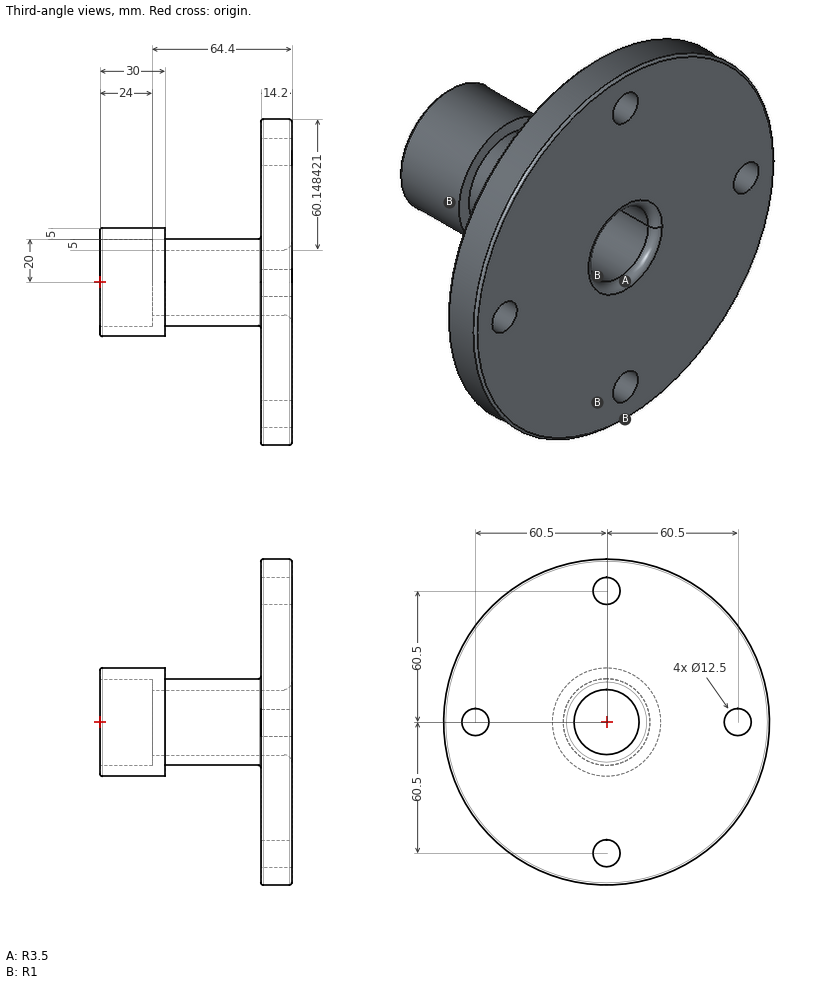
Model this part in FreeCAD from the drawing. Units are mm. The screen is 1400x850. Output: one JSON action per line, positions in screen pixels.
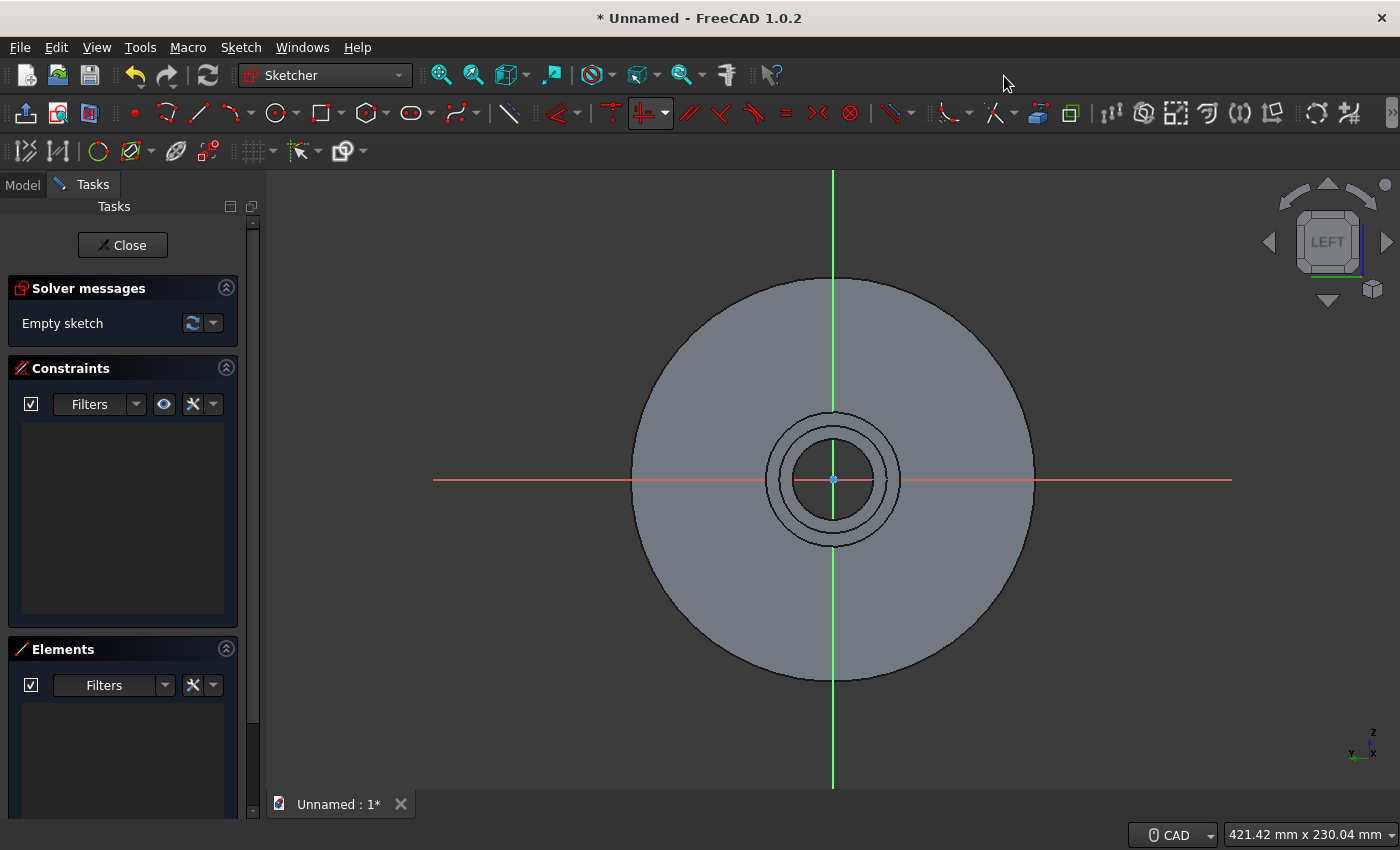
{"action": "key", "text": "q s"}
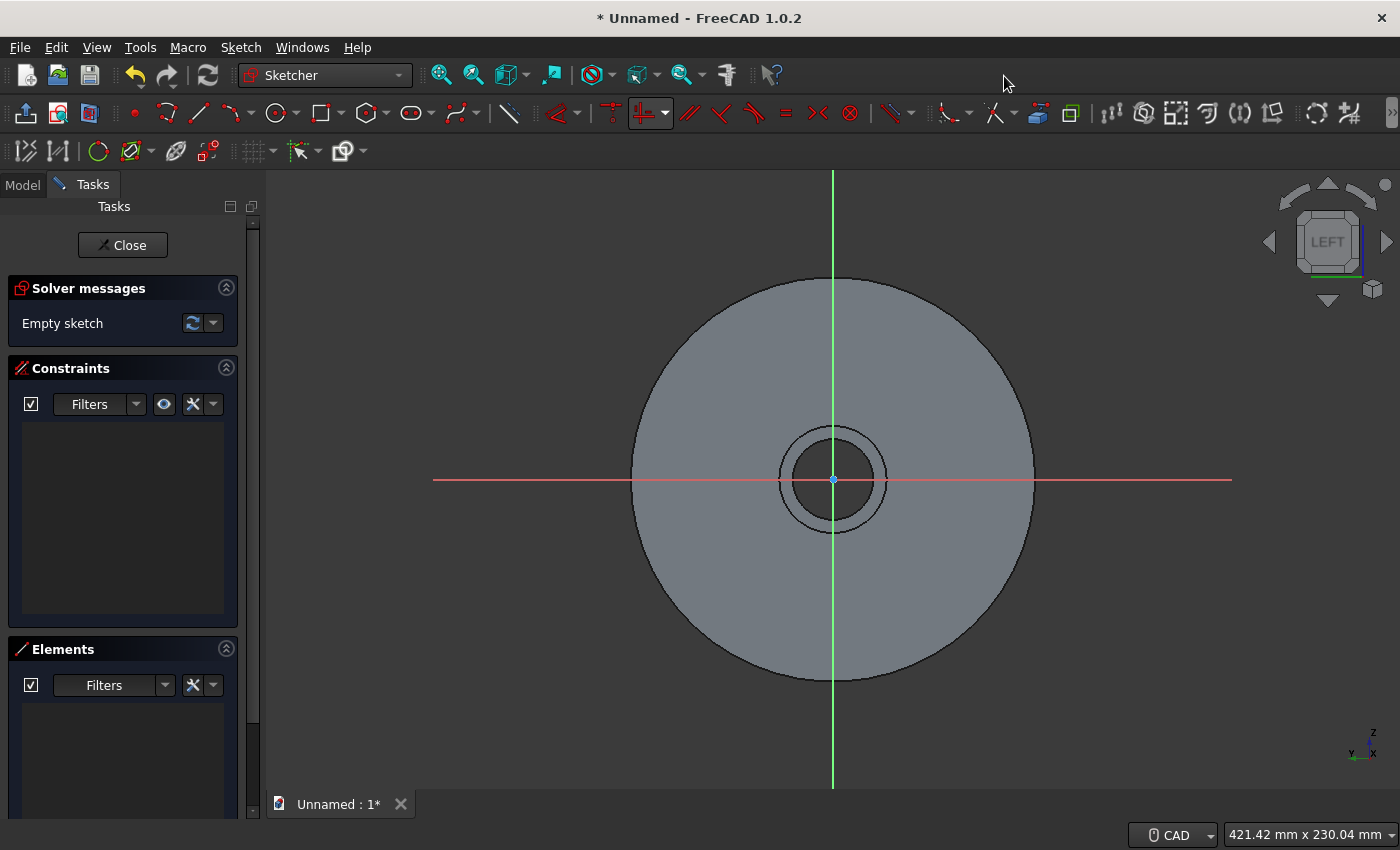
{"action": "key", "text": "g c"}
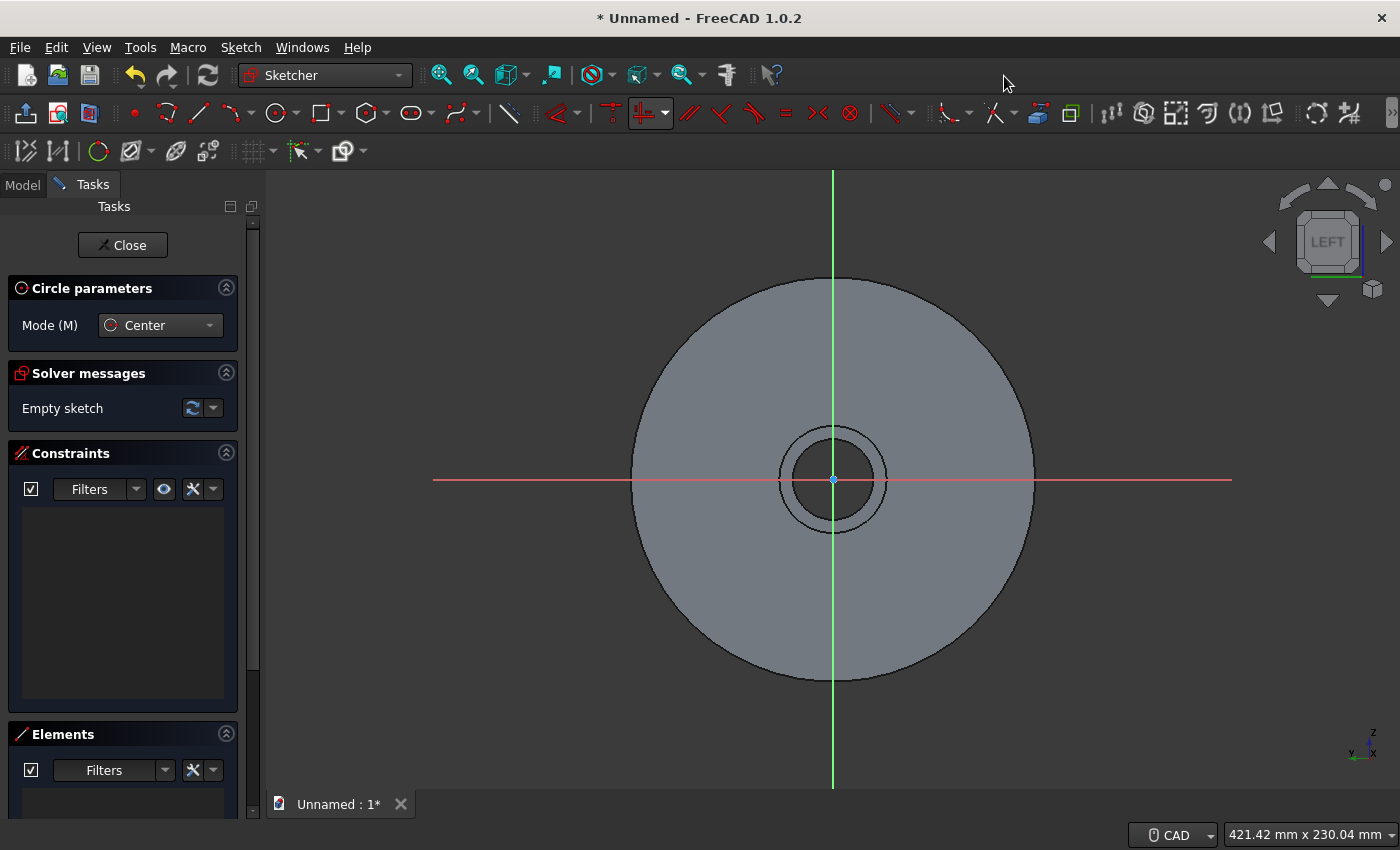
{"action": "scroll", "coordinate": [670, 480], "scroll_direction": "up", "scroll_amount": 2}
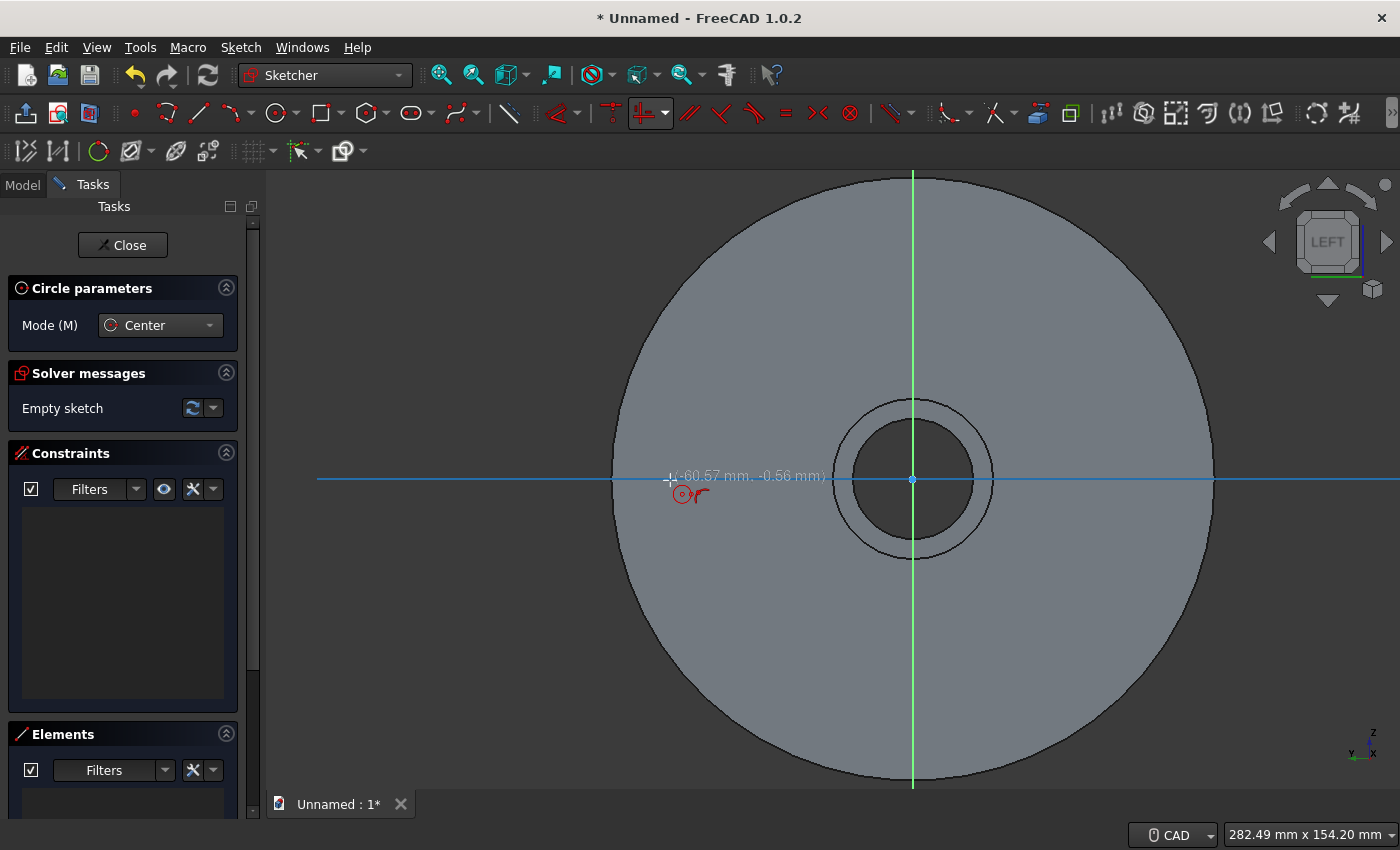
{"action": "left_click", "coordinate": [670, 479]}
{"action": "mouse_move", "coordinate": [688, 461]}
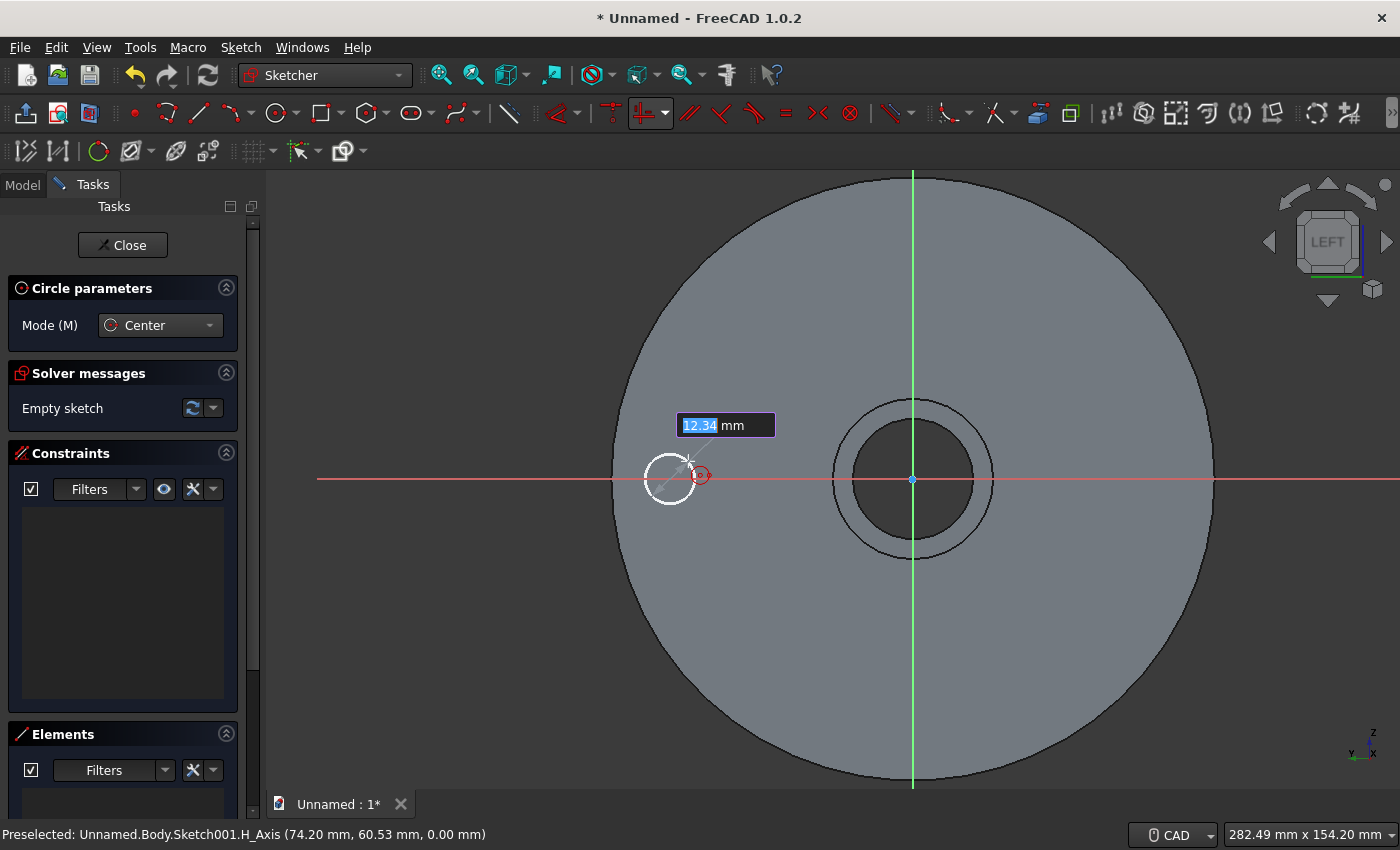
{"action": "type", "text": "12.5"}
{"action": "key", "text": "Return"}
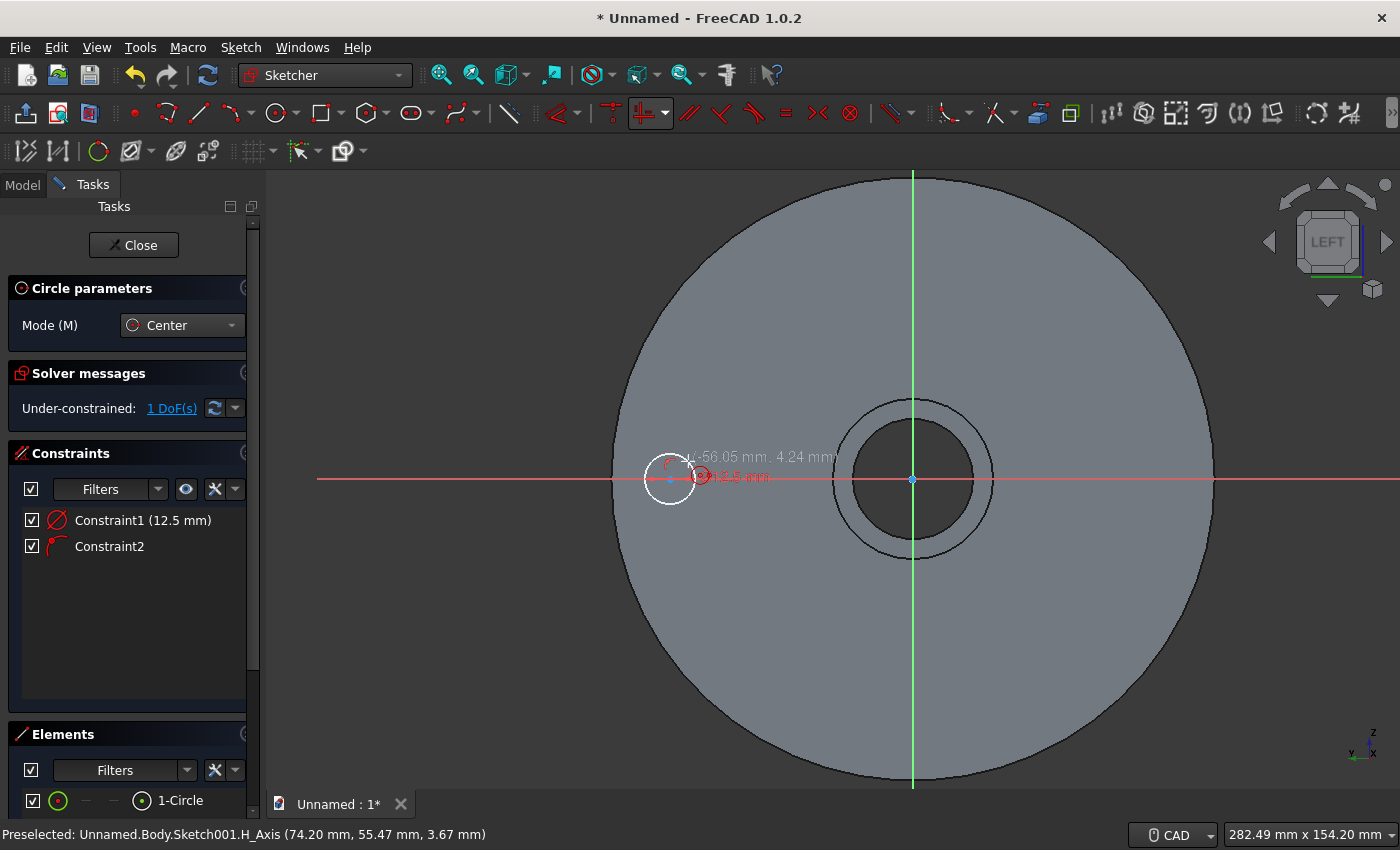
{"action": "left_click", "coordinate": [1156, 479]}
{"action": "mouse_move", "coordinate": [1174, 461]}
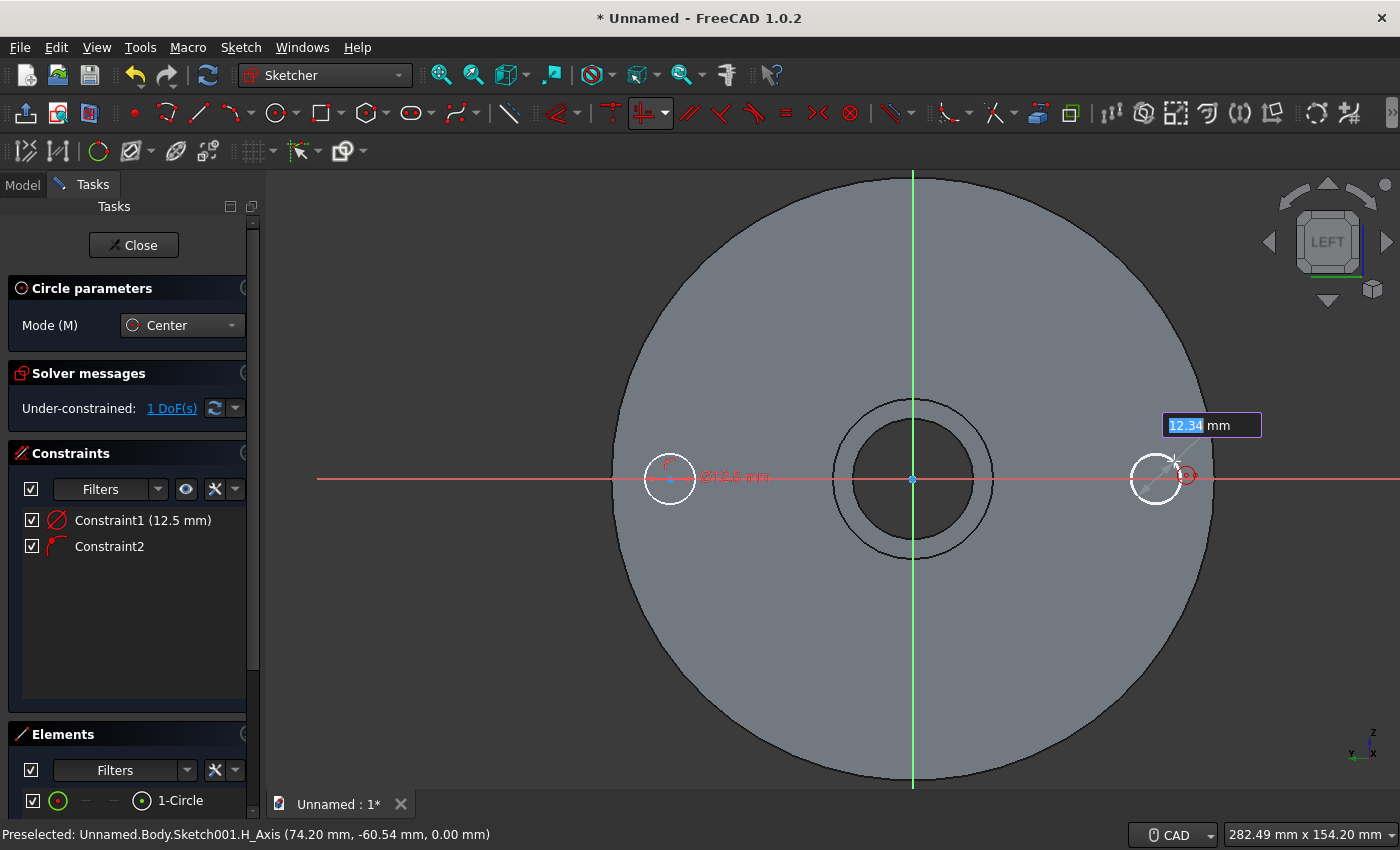
{"action": "type", "text": "12.5"}
{"action": "key", "text": "Return"}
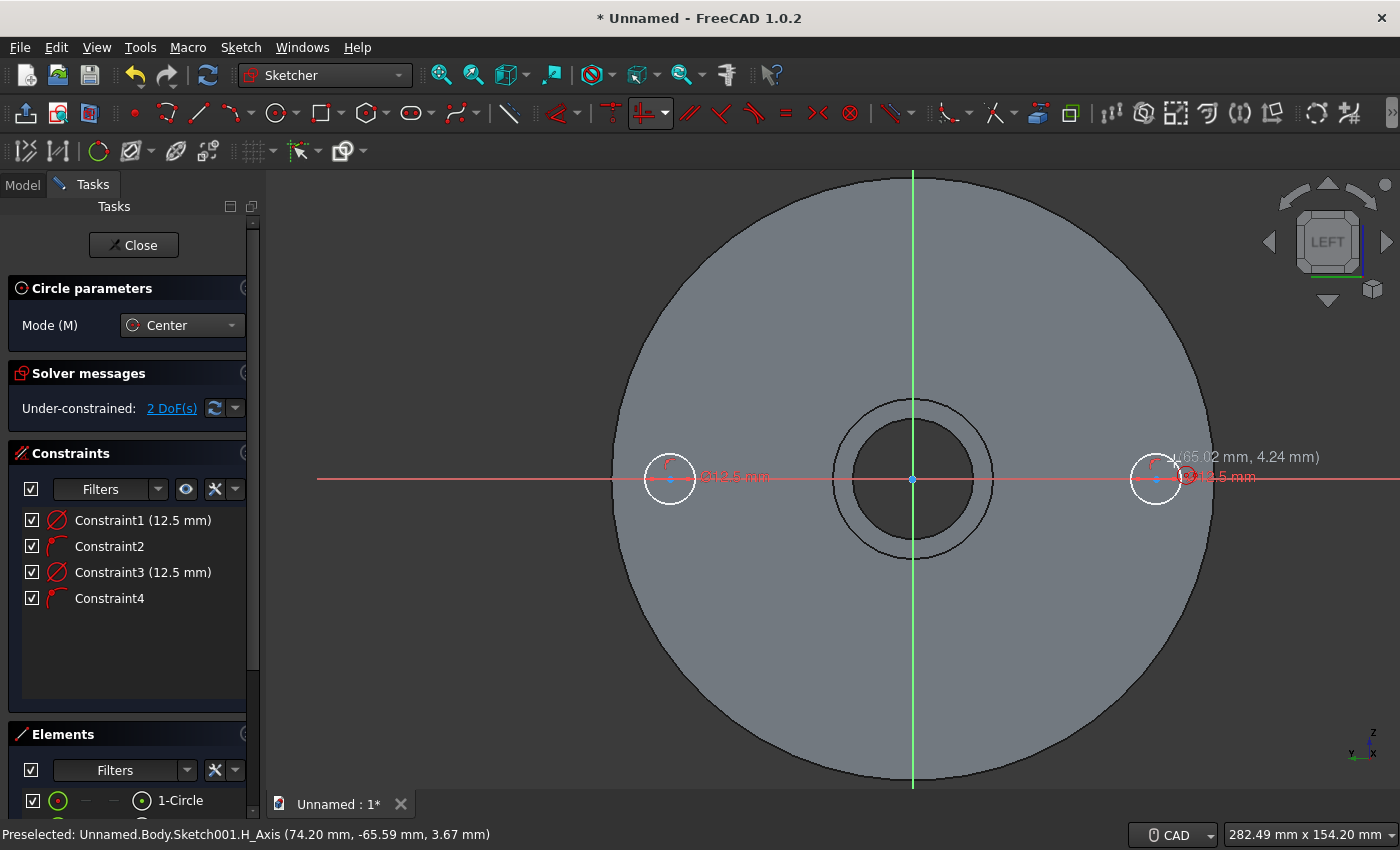
{"action": "left_click", "coordinate": [913, 722]}
{"action": "mouse_move", "coordinate": [931, 704]}